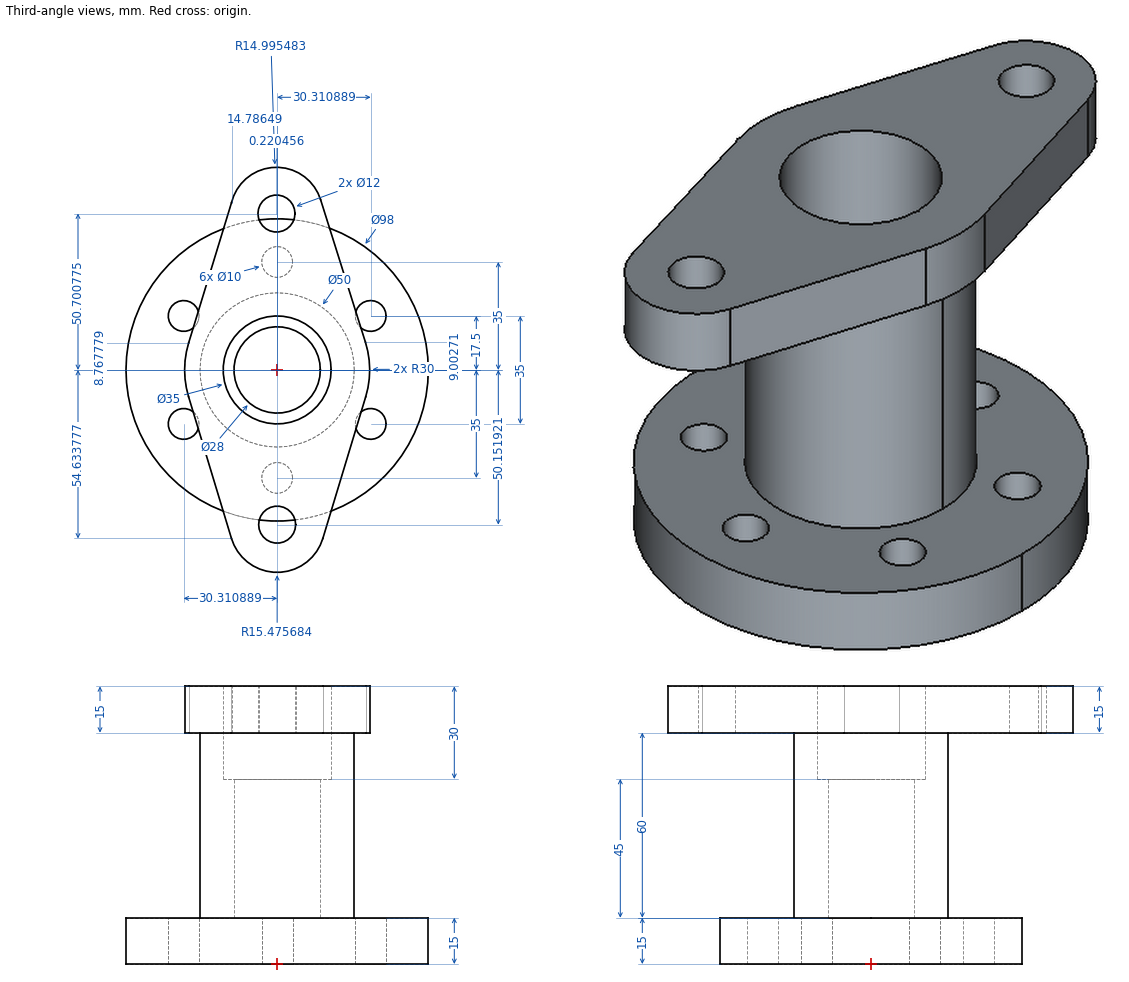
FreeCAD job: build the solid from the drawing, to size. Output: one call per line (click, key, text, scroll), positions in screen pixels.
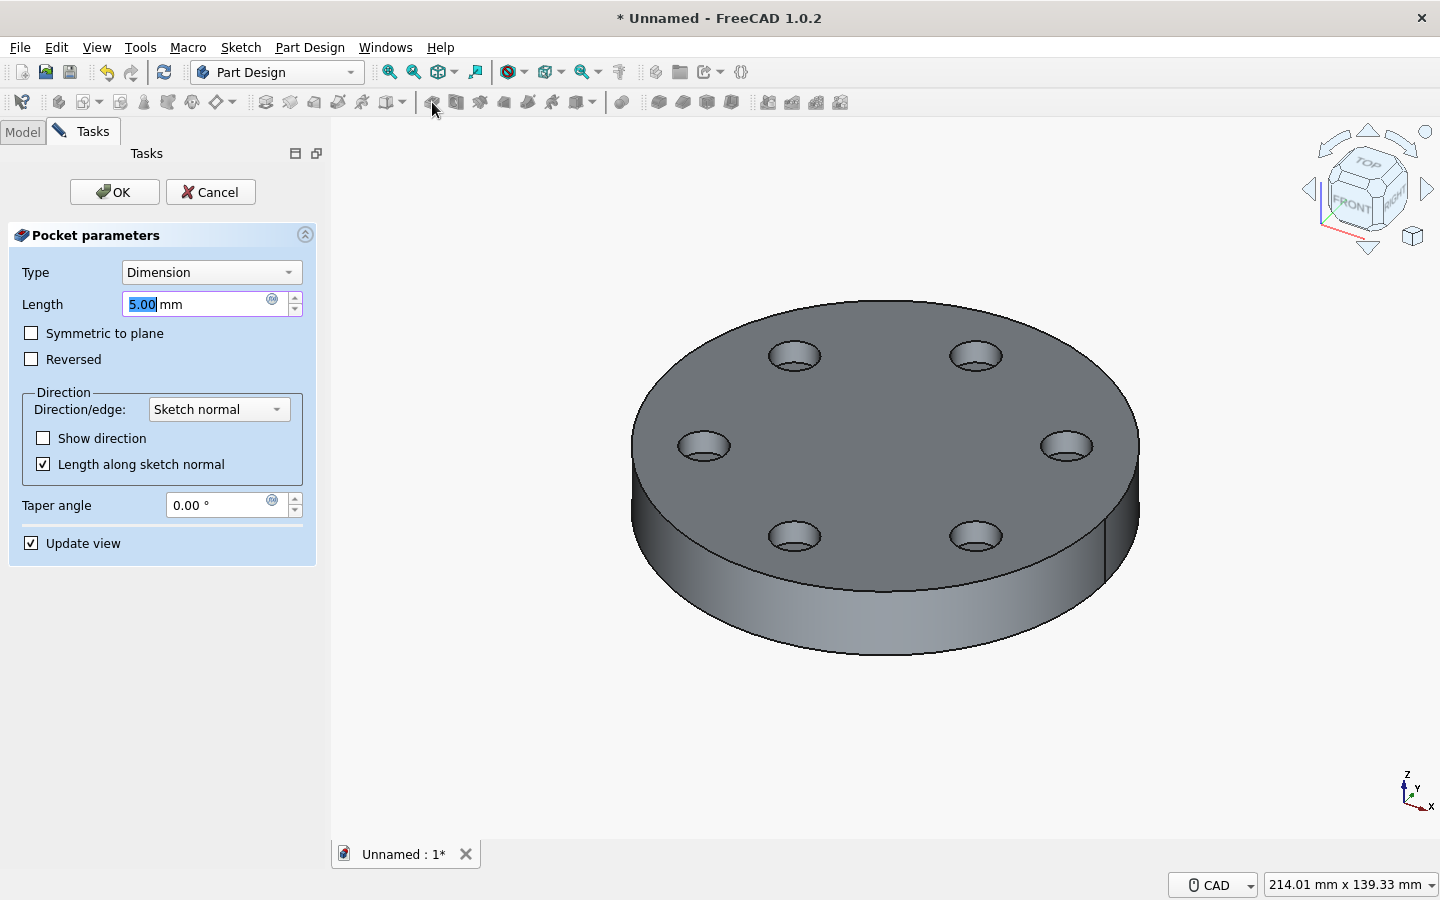
text(15)
key(Tab)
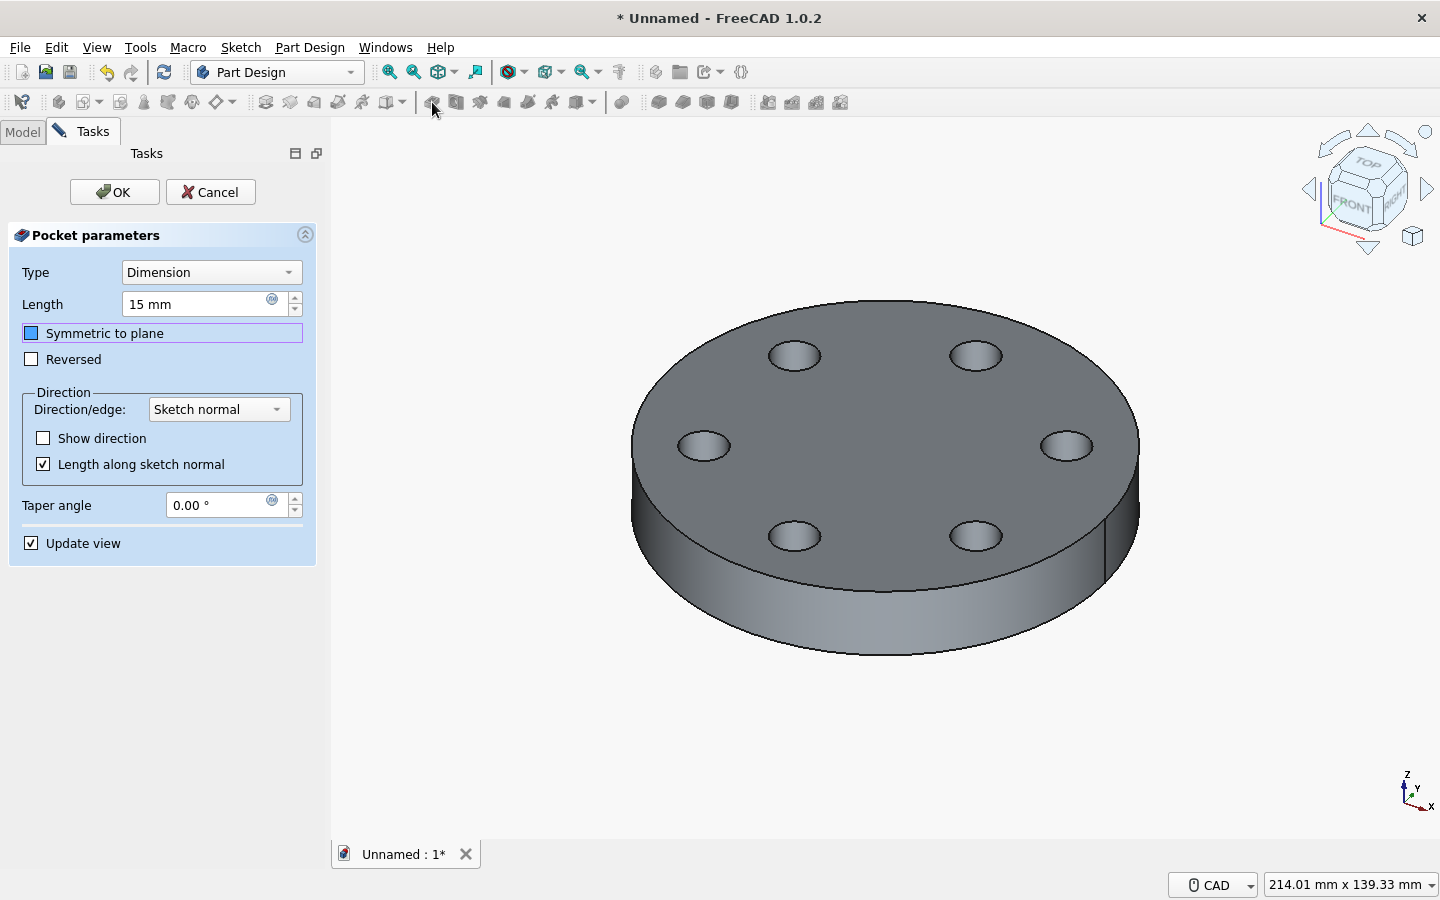
click(115, 192)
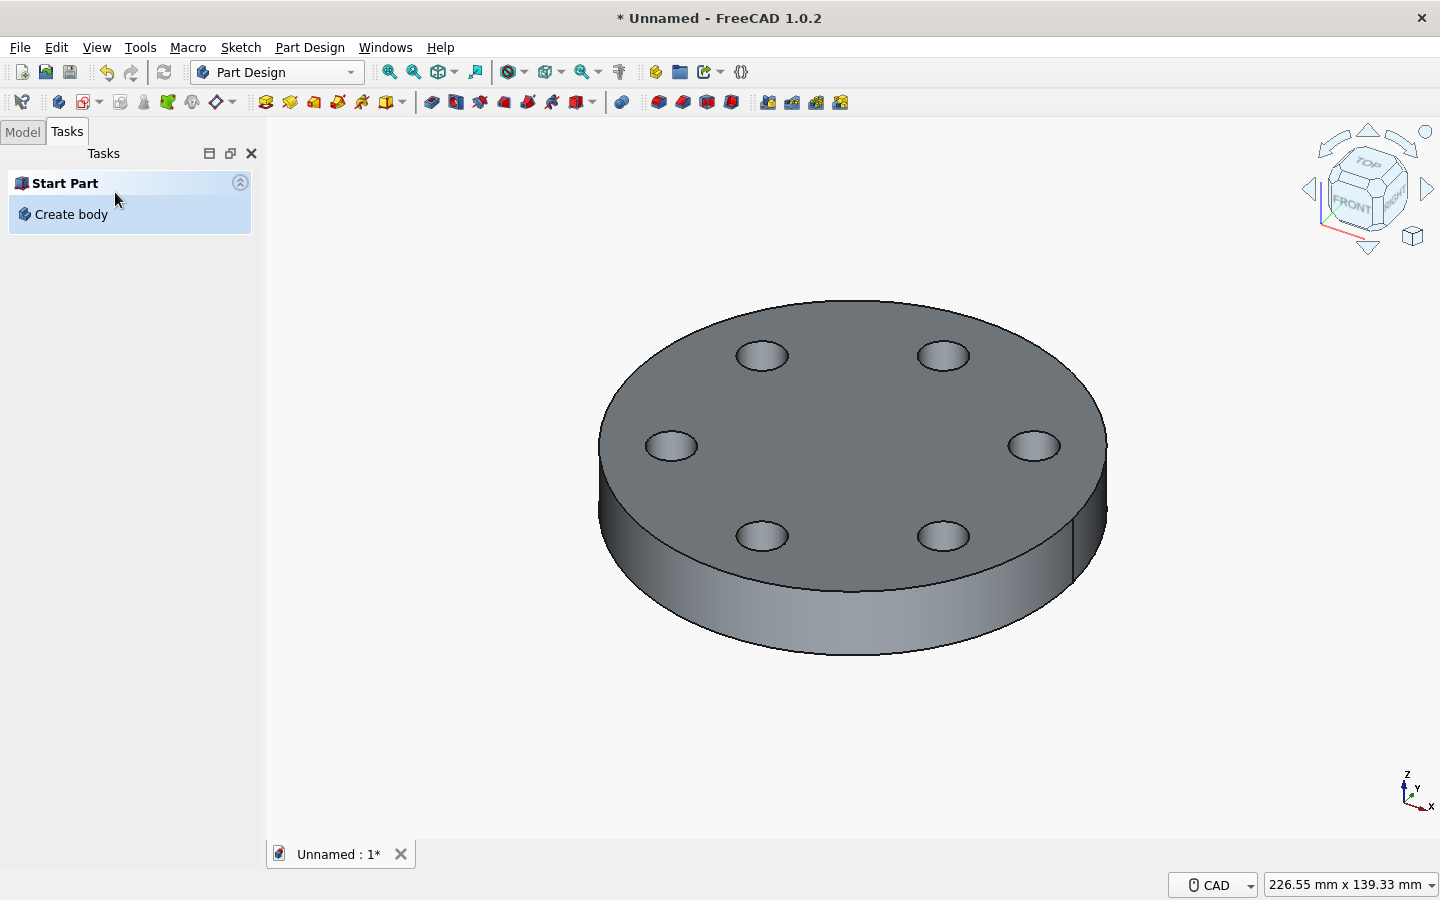
click(853, 445)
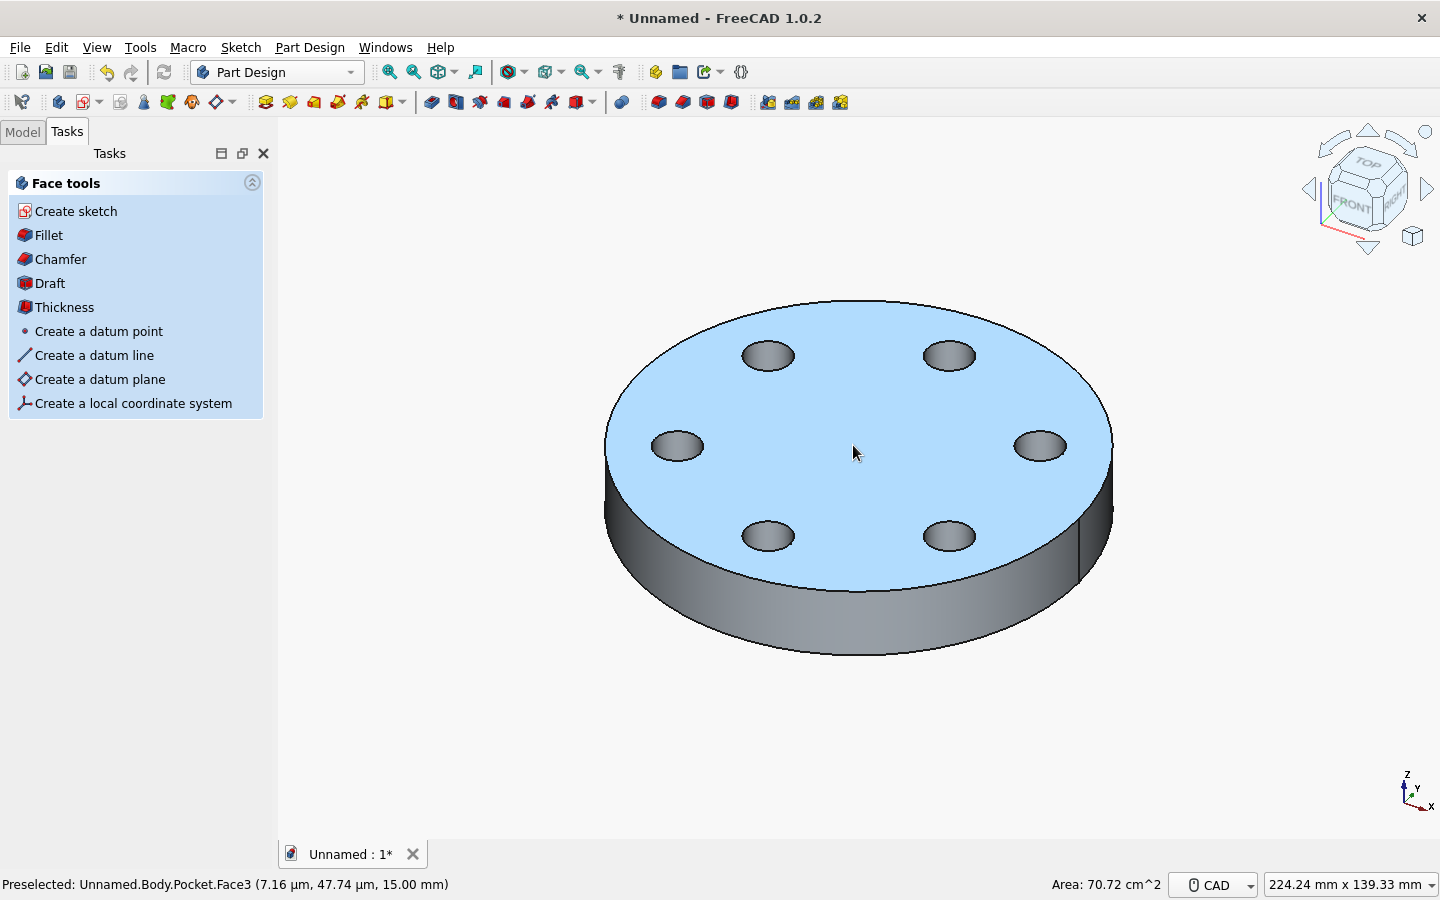
click(84, 102)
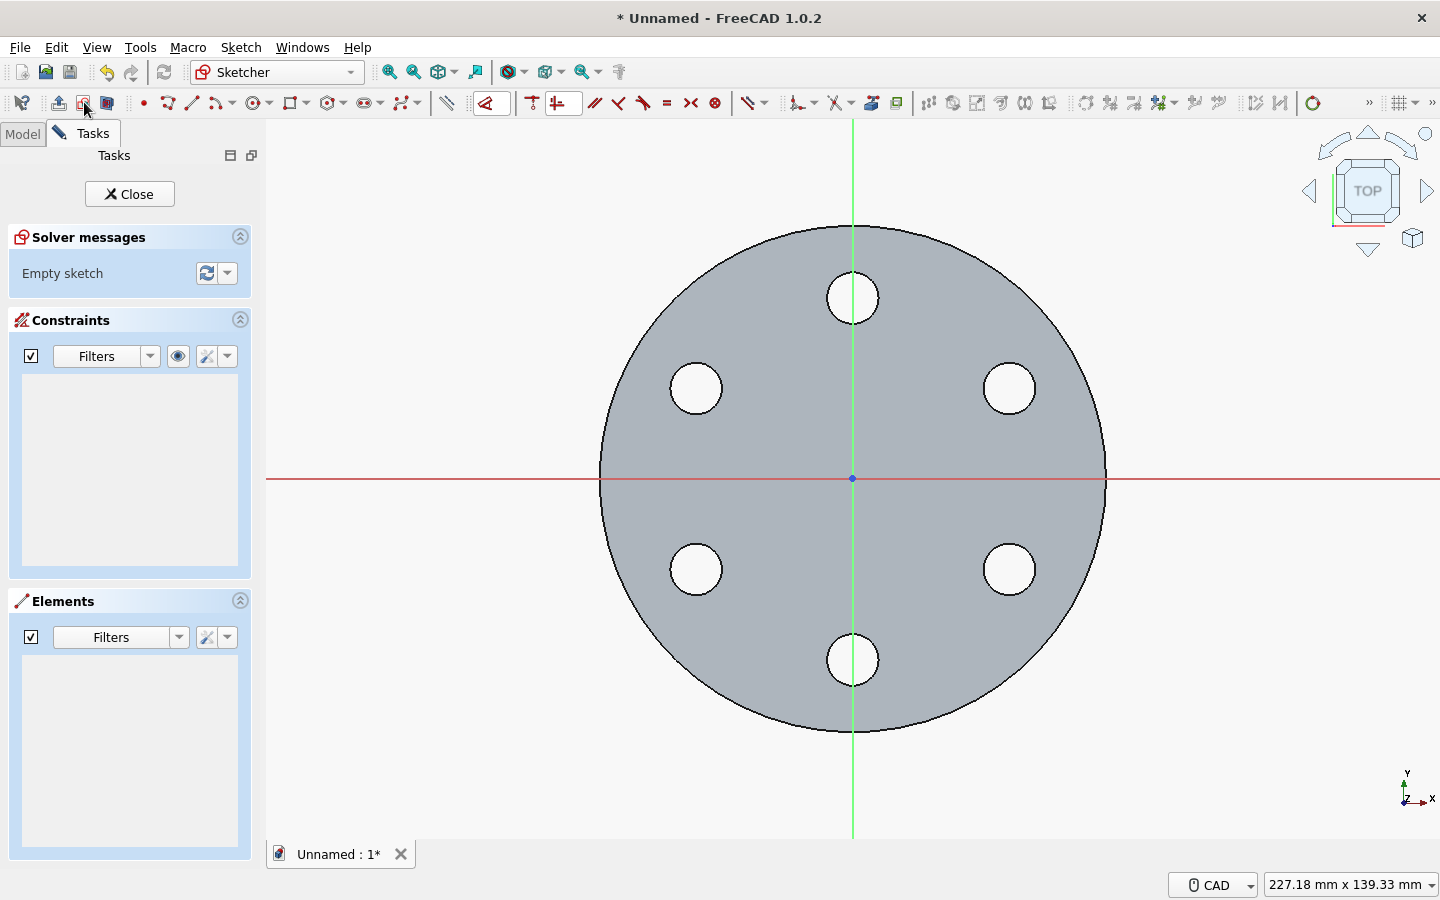
scroll(936, 479, up, 3)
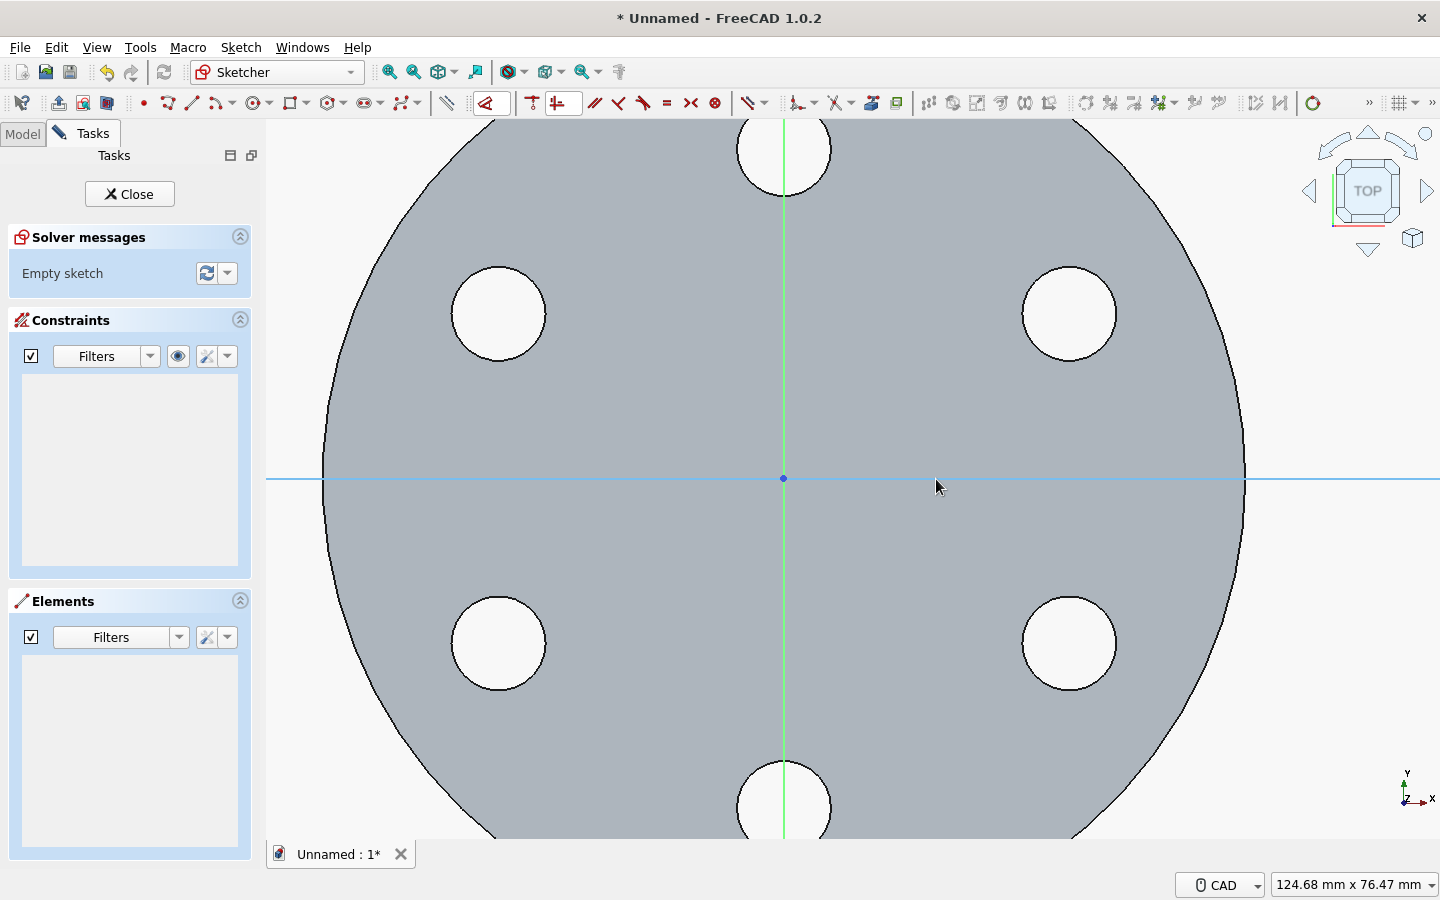
click(254, 104)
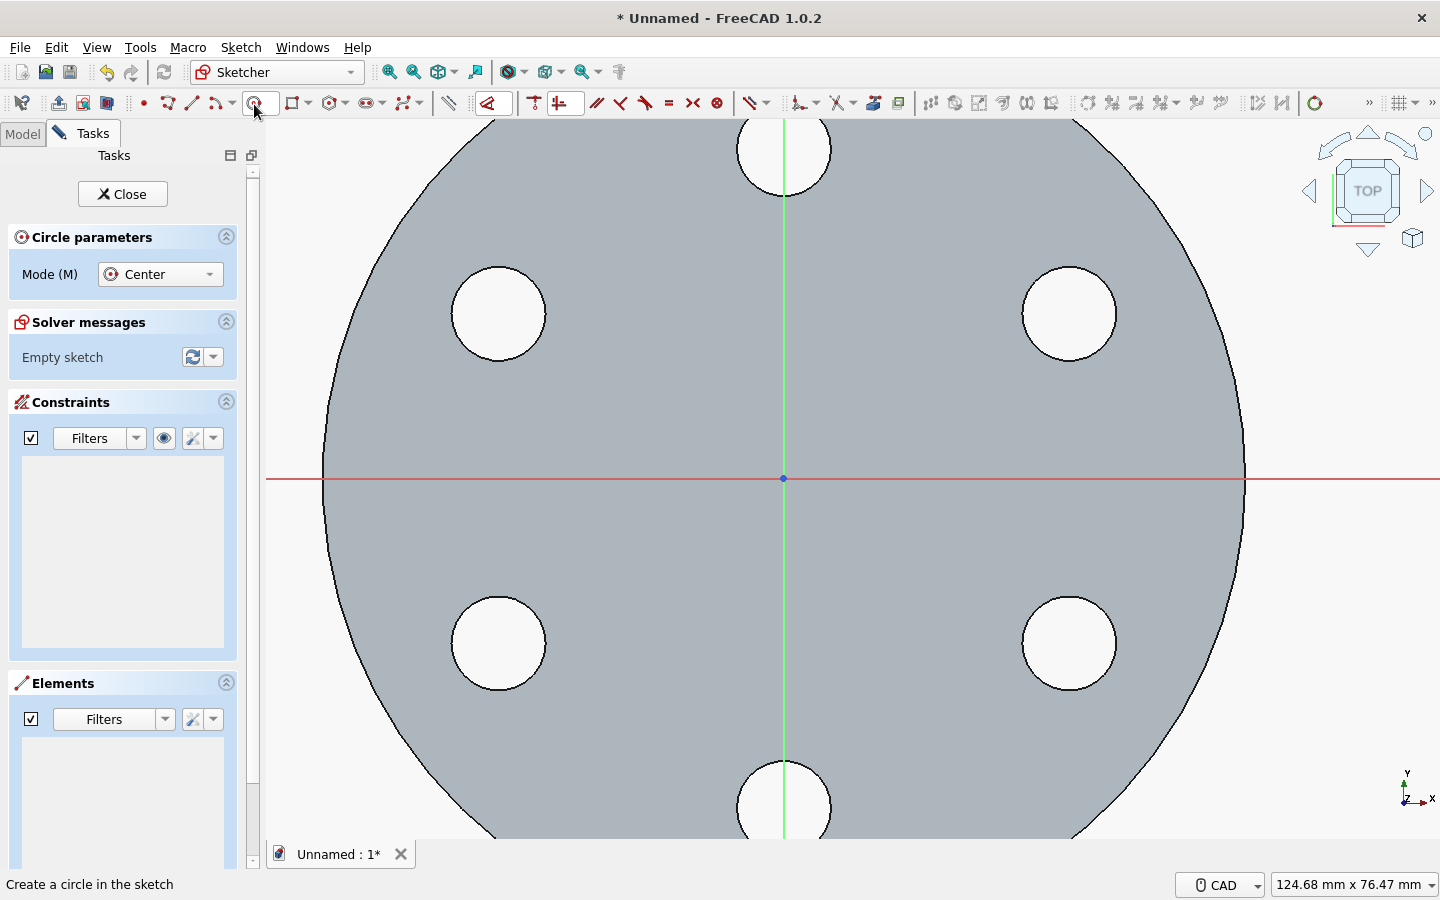
click(784, 479)
click(950, 312)
key(Escape)